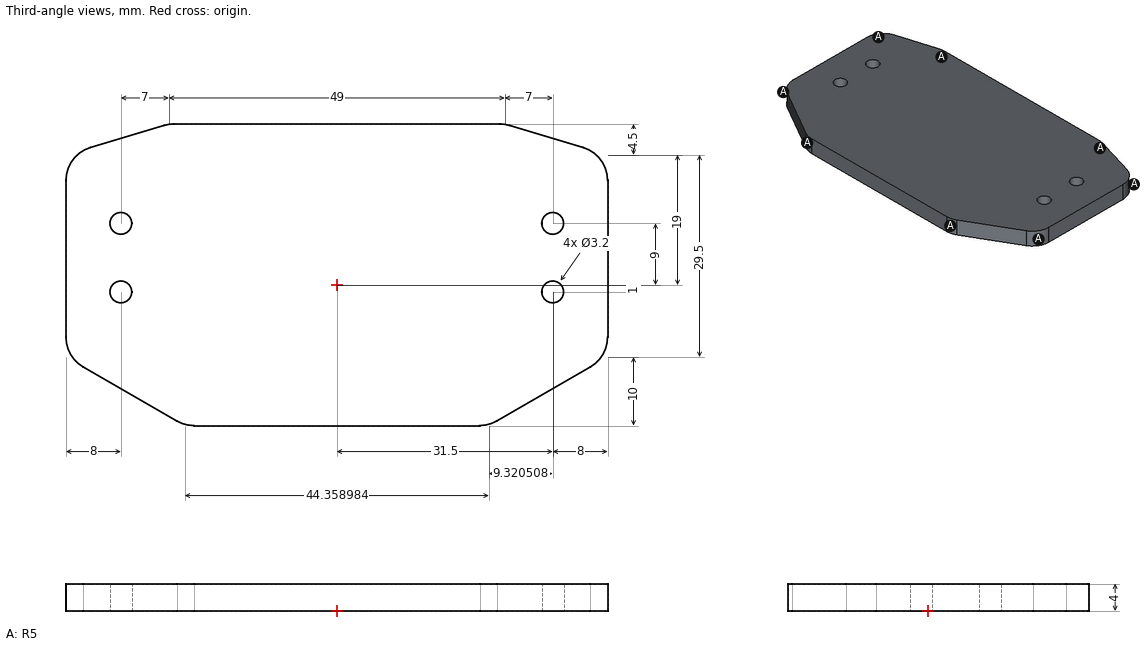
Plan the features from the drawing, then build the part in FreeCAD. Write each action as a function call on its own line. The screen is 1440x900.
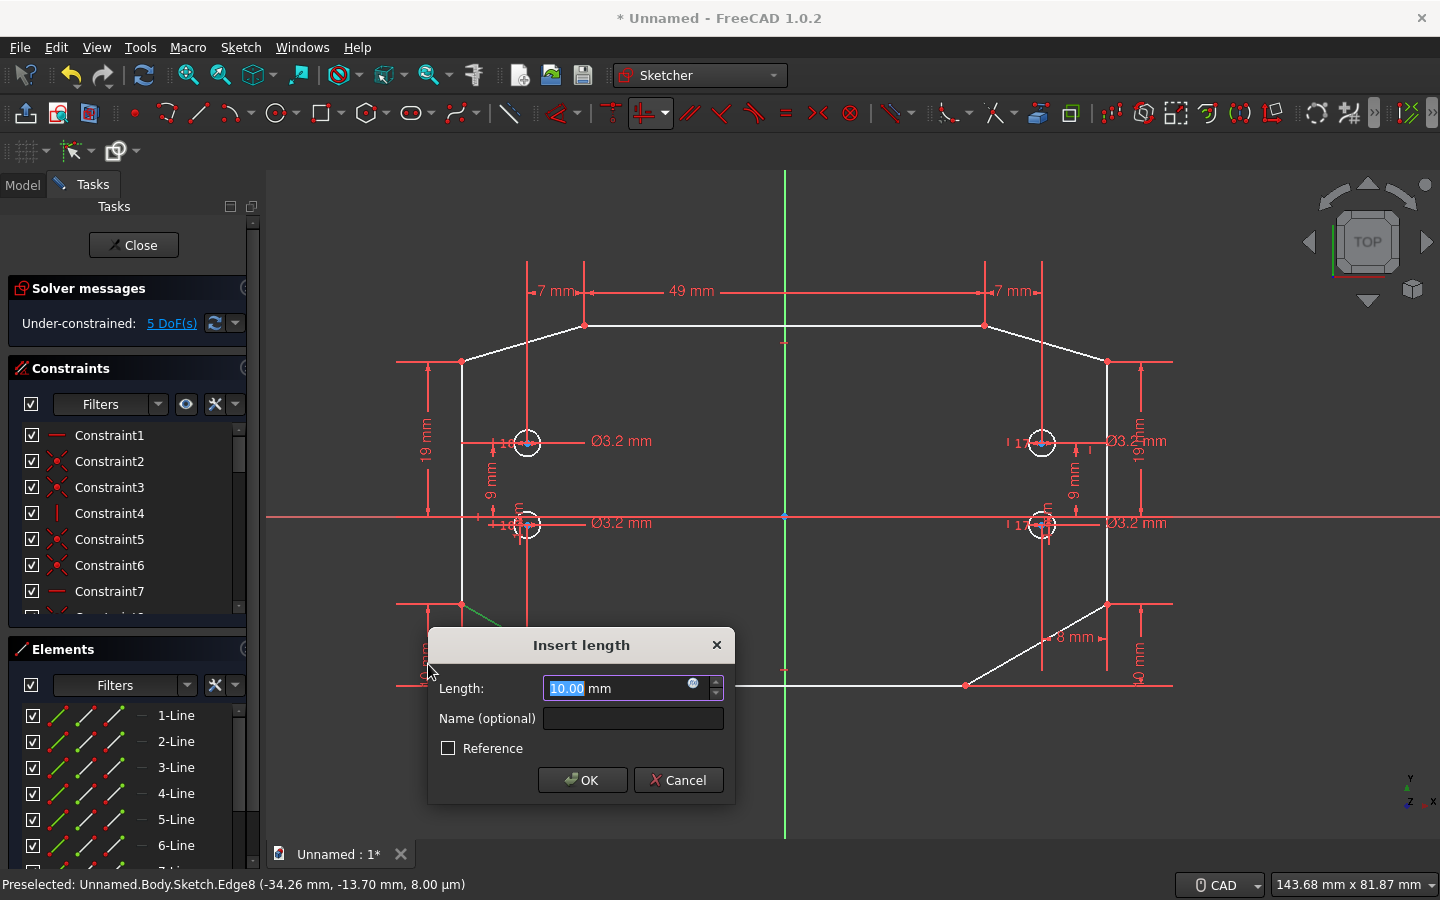
text(10)
key(Return)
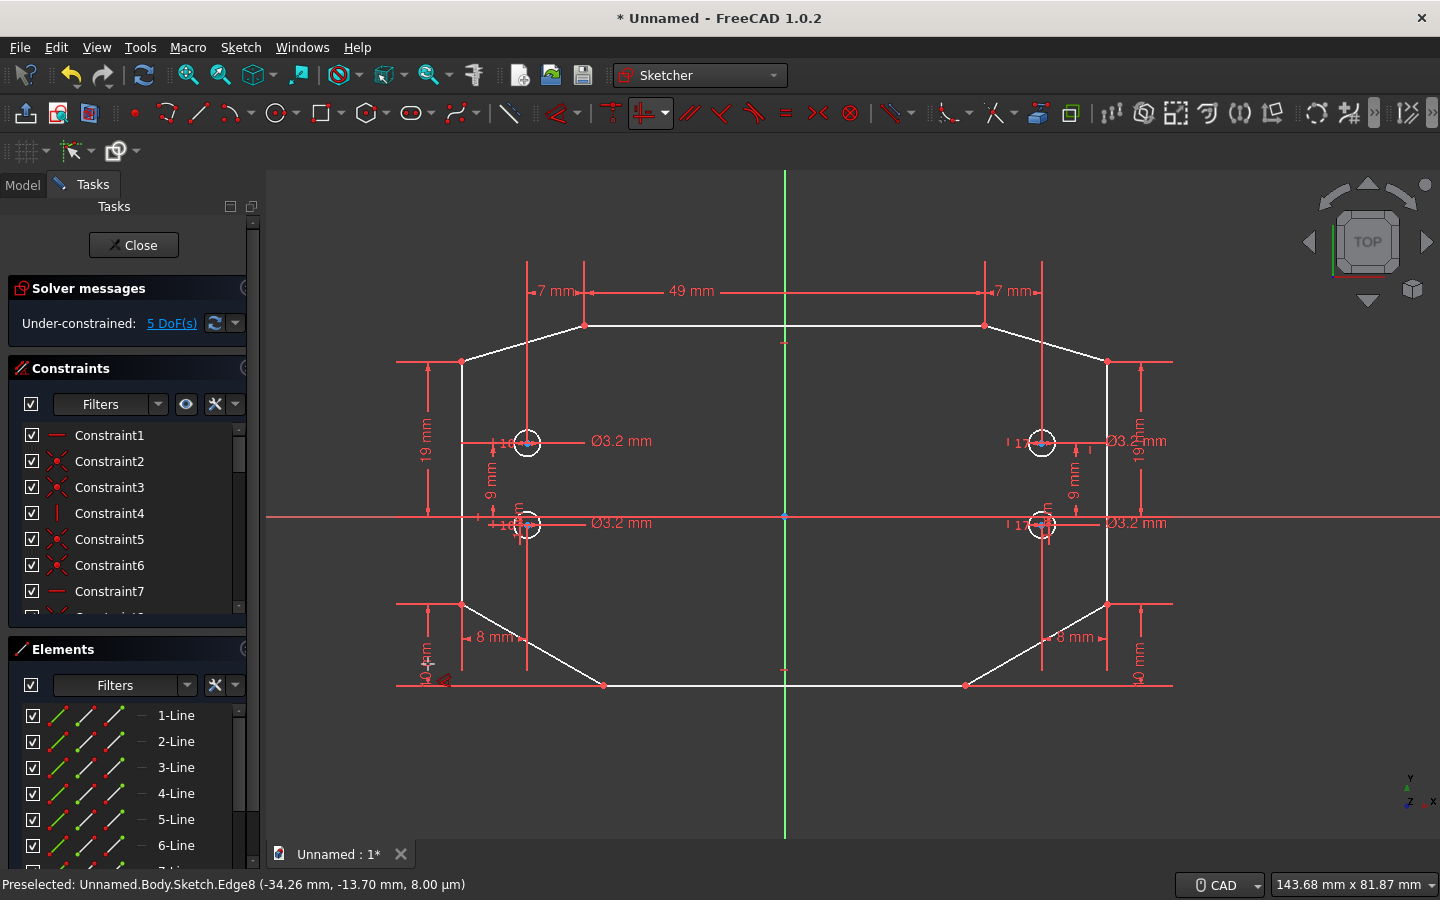
click(1107, 531)
click(1141, 539)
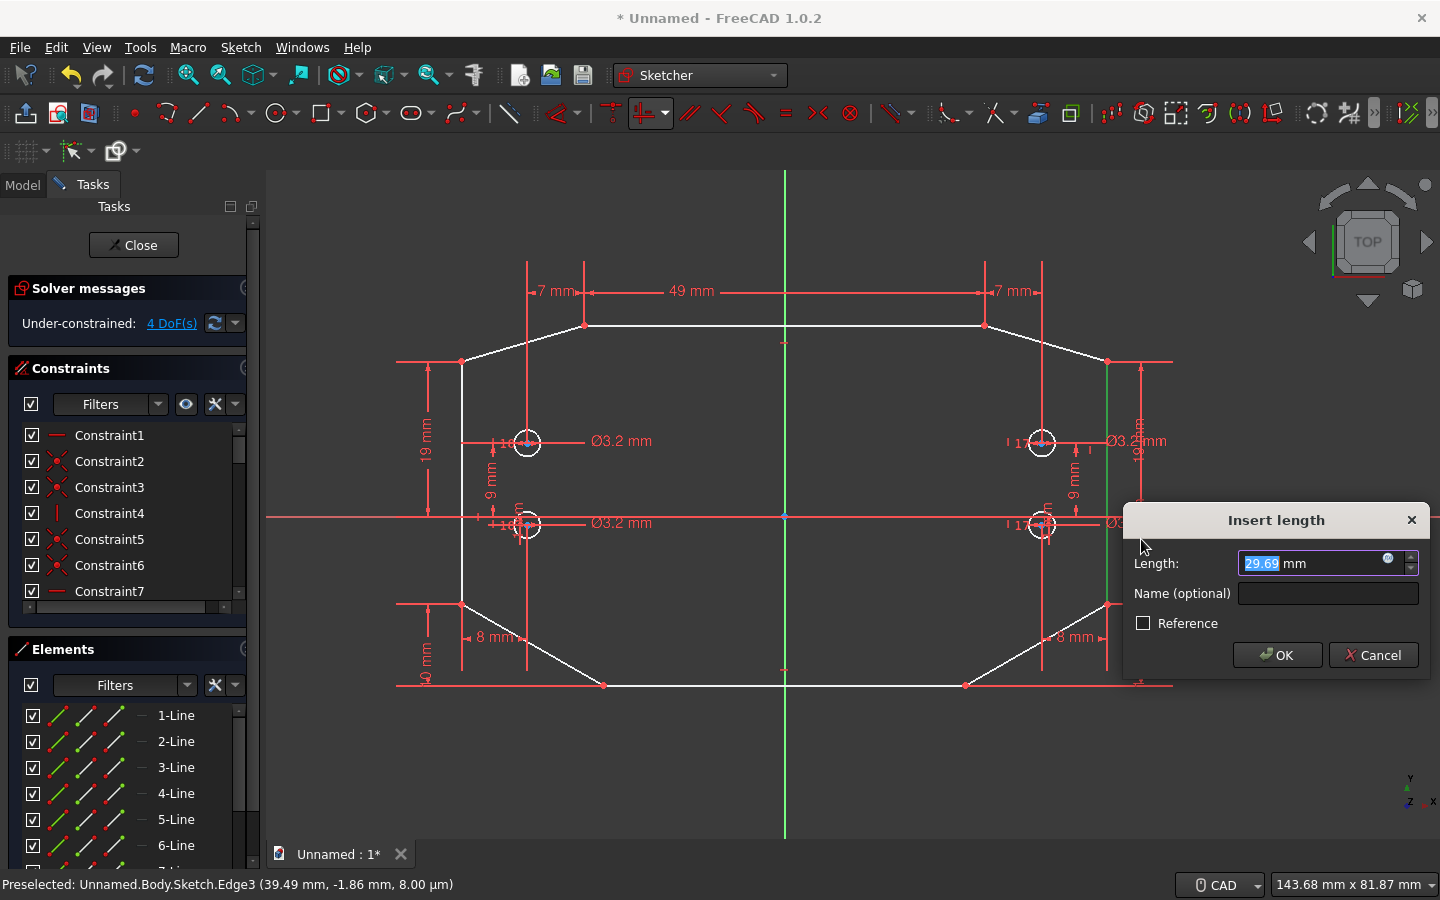
text(29.5)
key(Return)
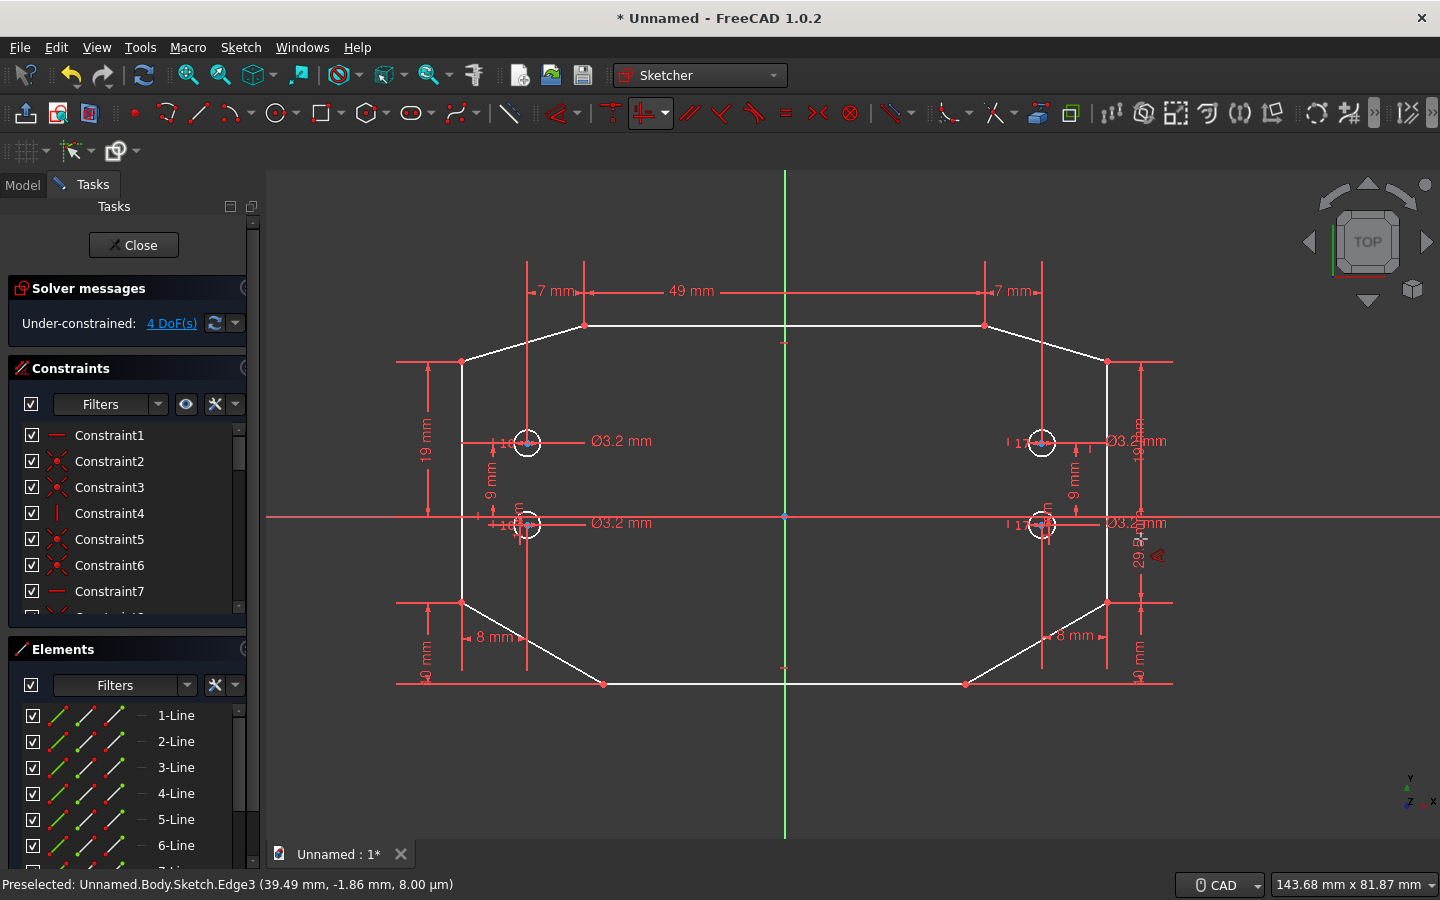
click(1071, 351)
click(1141, 344)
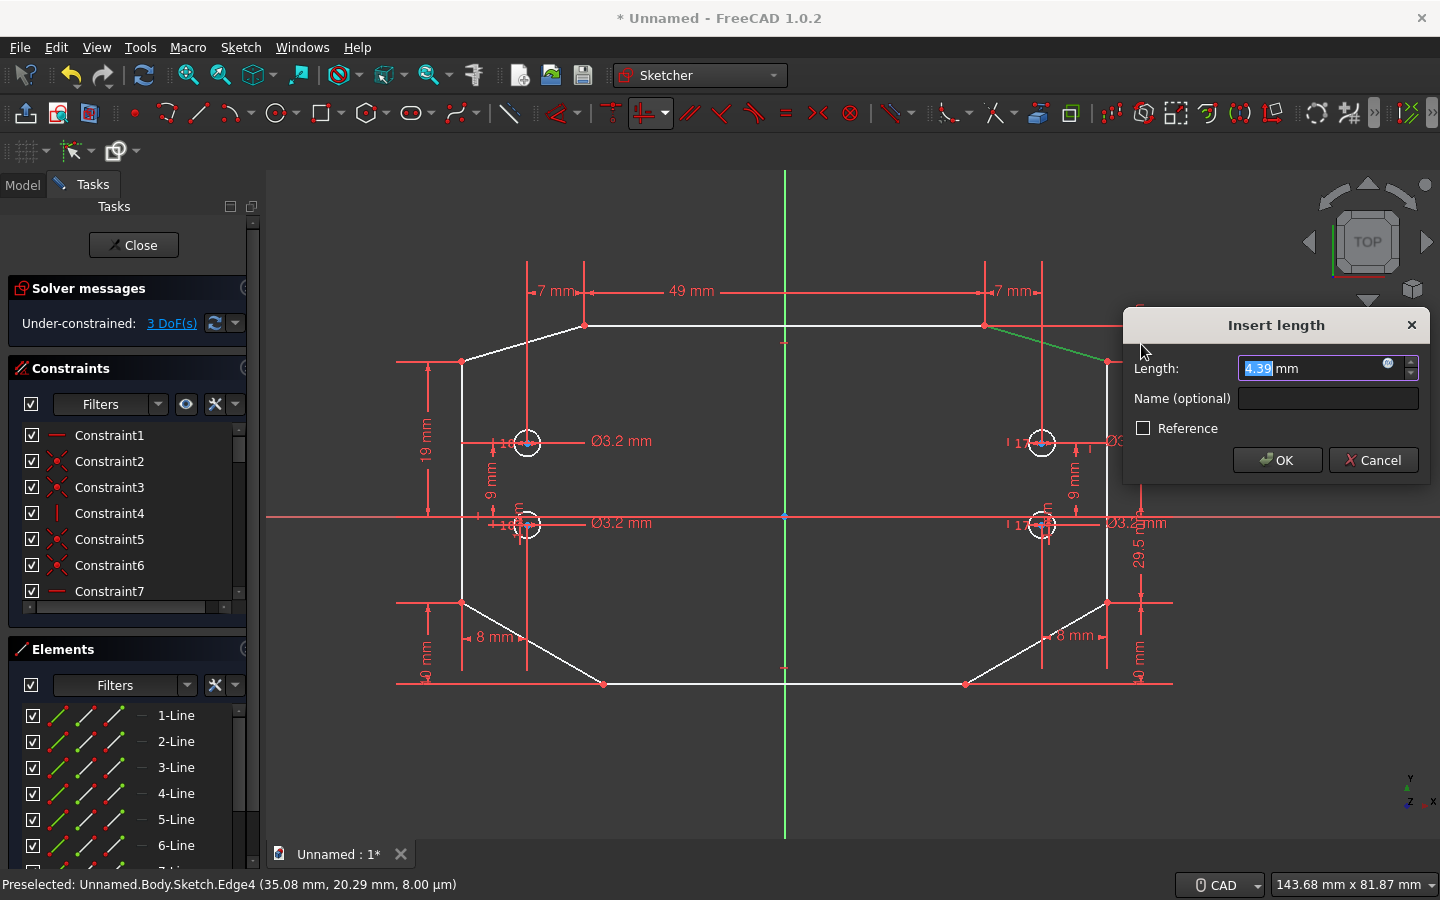
text(4.5)
key(Return)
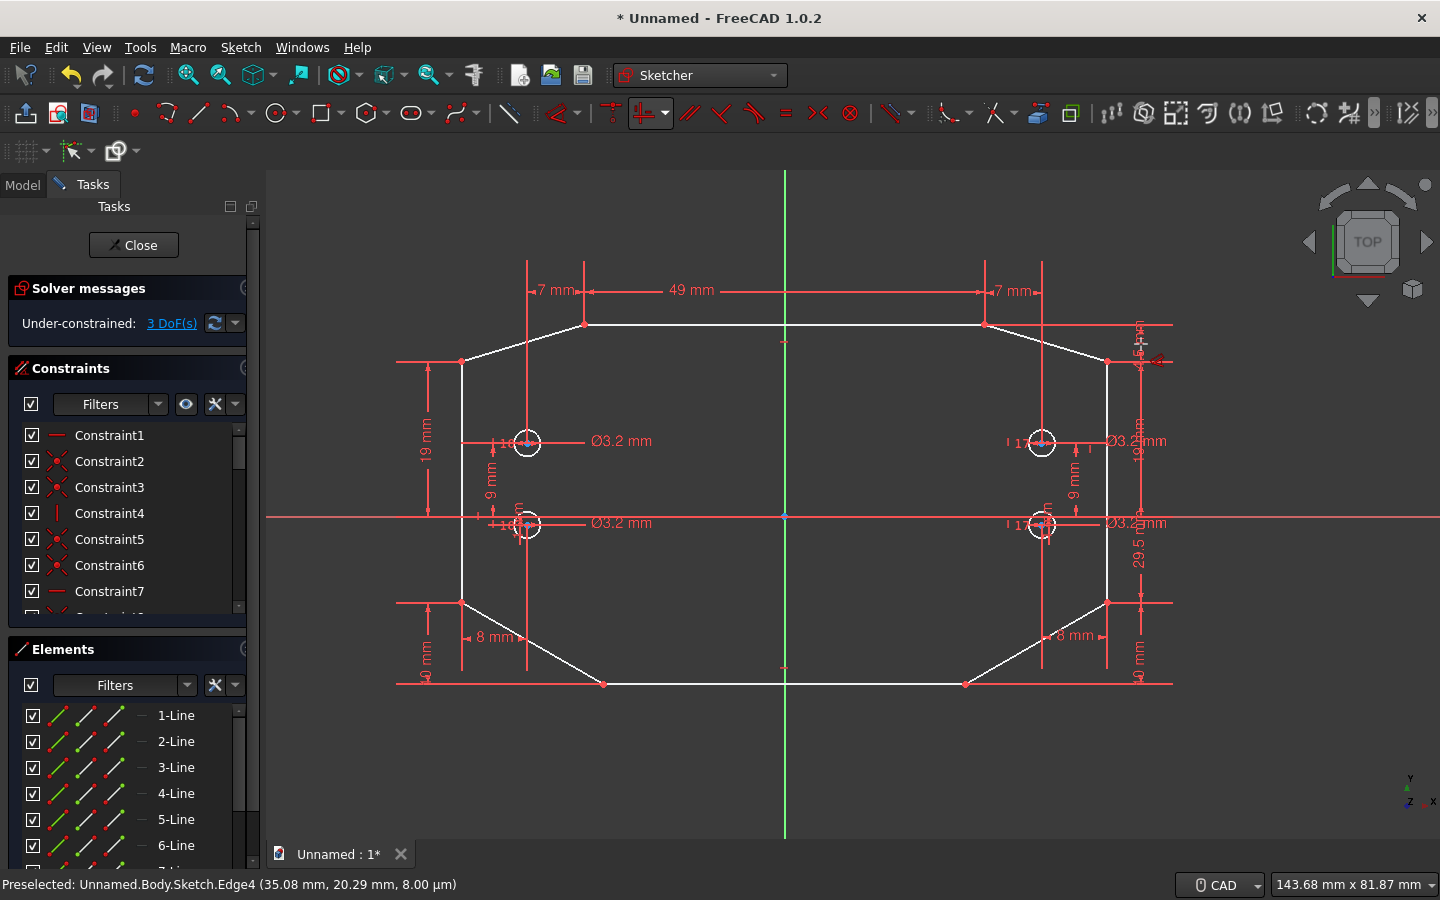
click(1042, 525)
click(913, 559)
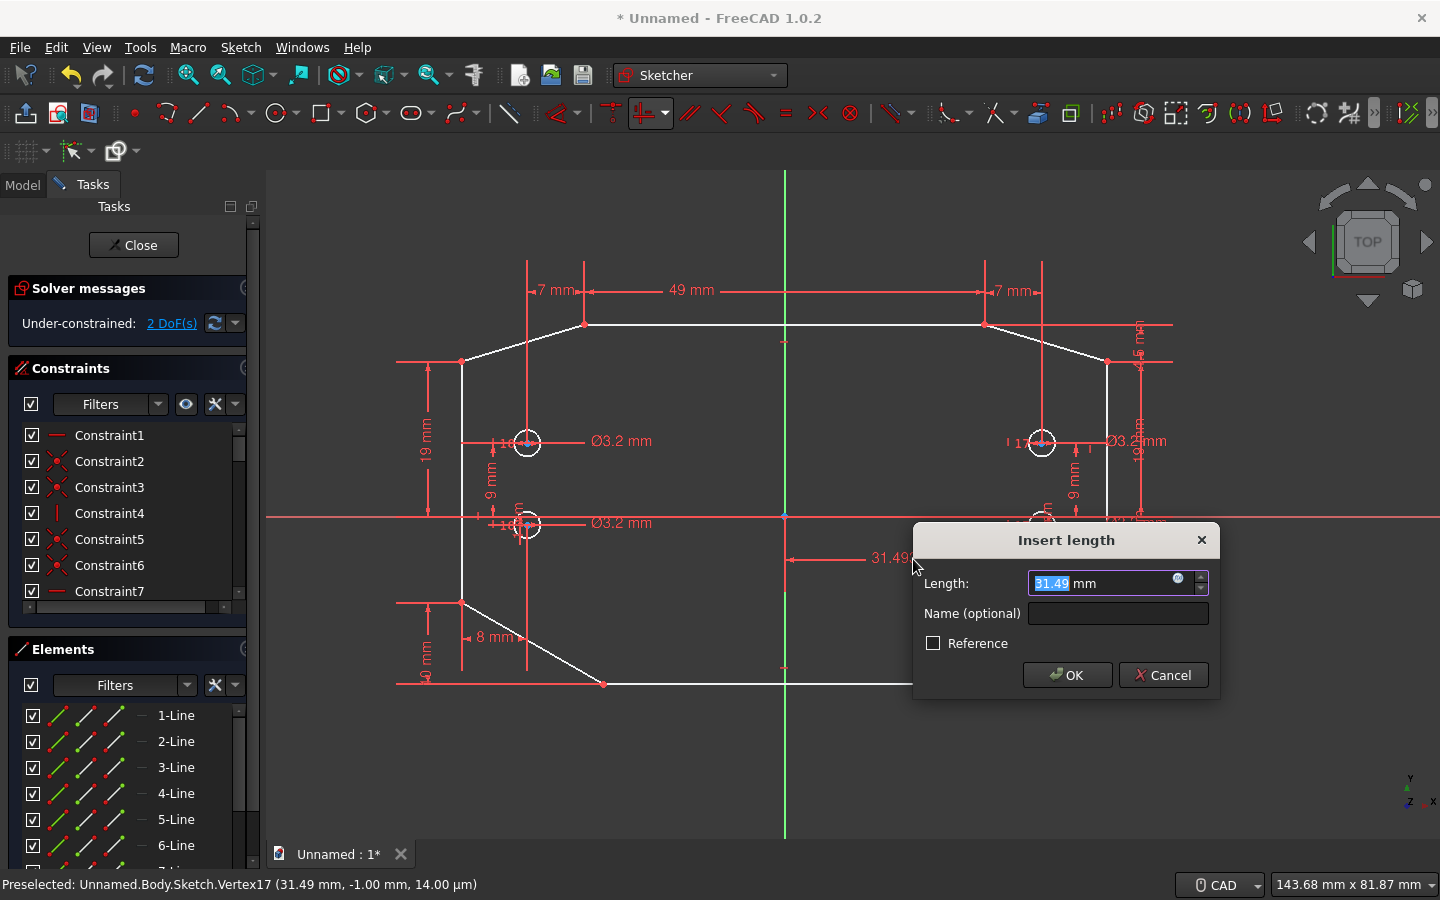
text(31.5)
key(Return)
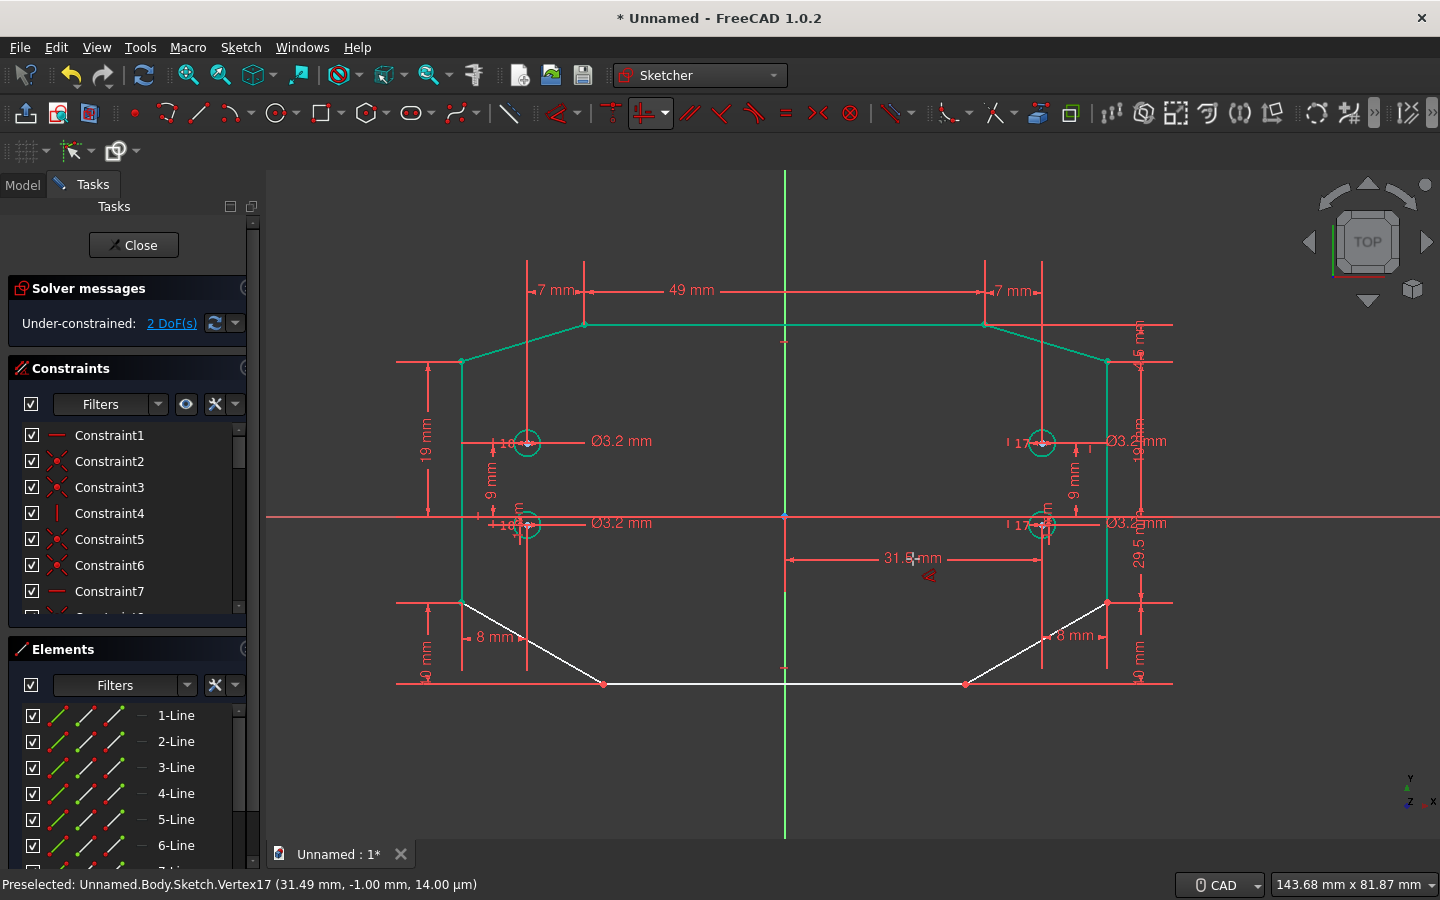
click(712, 684)
click(701, 718)